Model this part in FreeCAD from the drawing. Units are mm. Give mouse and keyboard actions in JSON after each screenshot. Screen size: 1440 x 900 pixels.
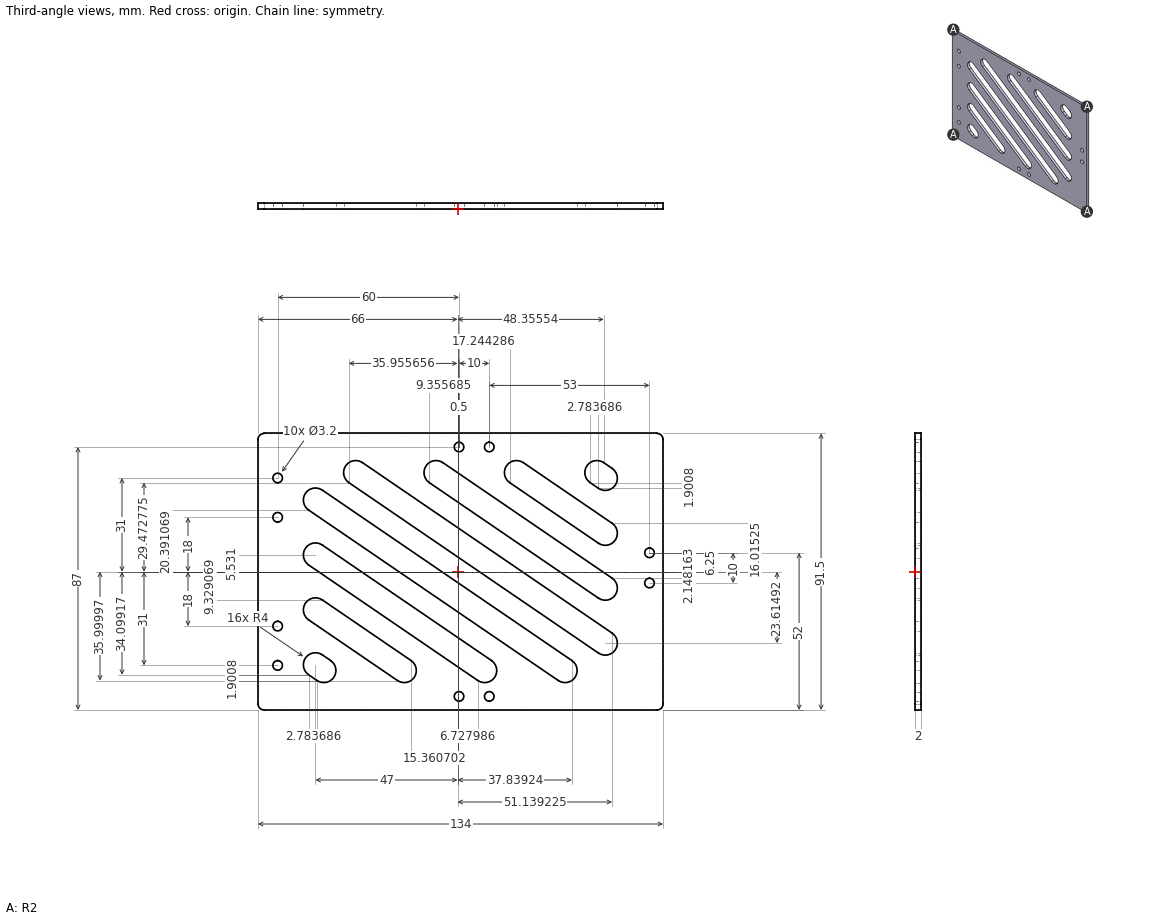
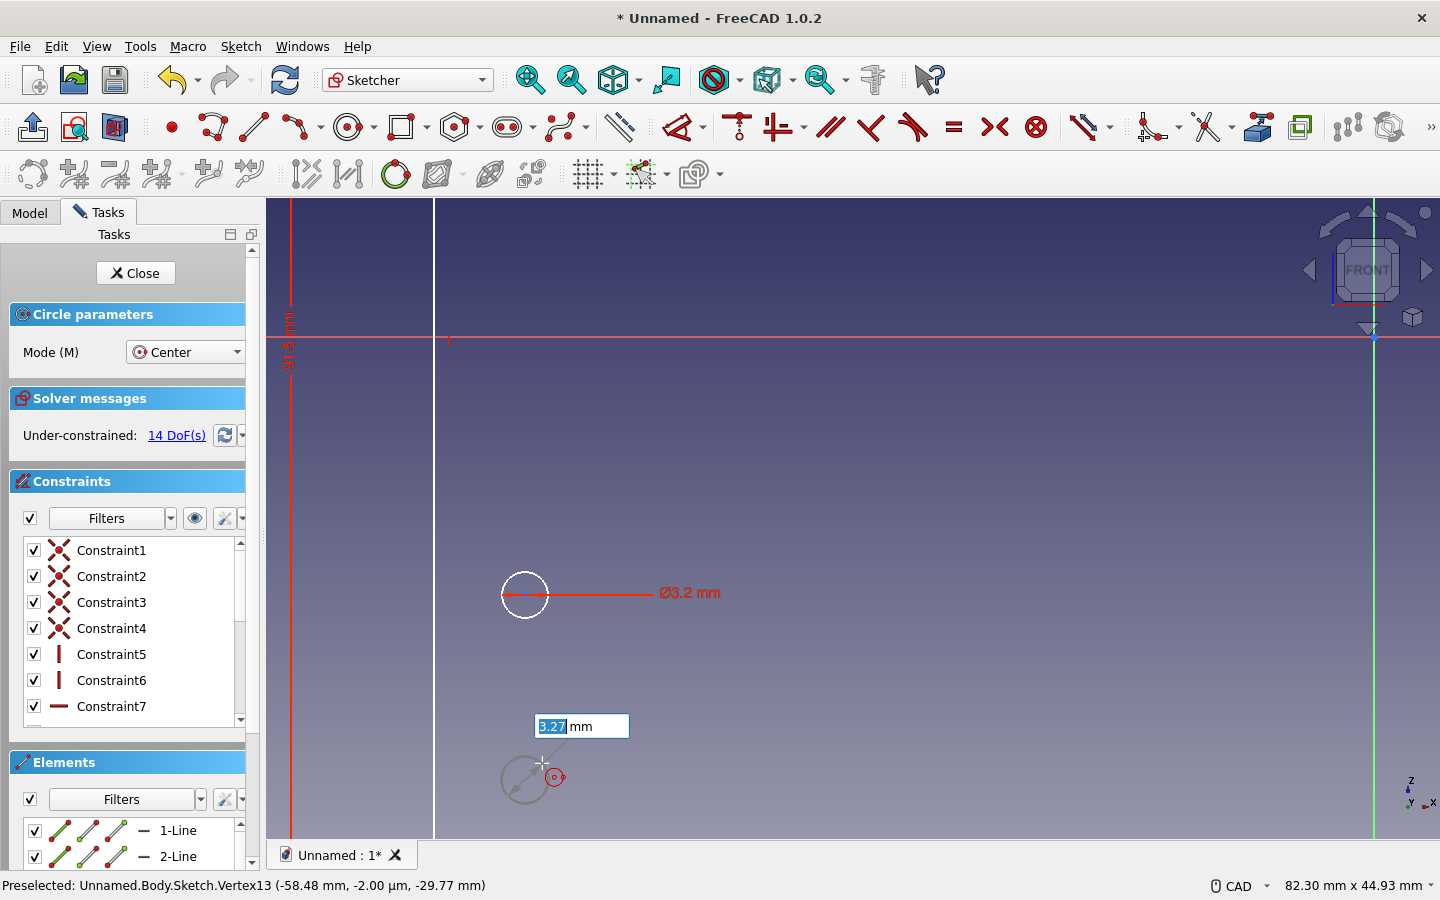
{"action": "type", "text": "3.2"}
{"action": "key", "text": "Return"}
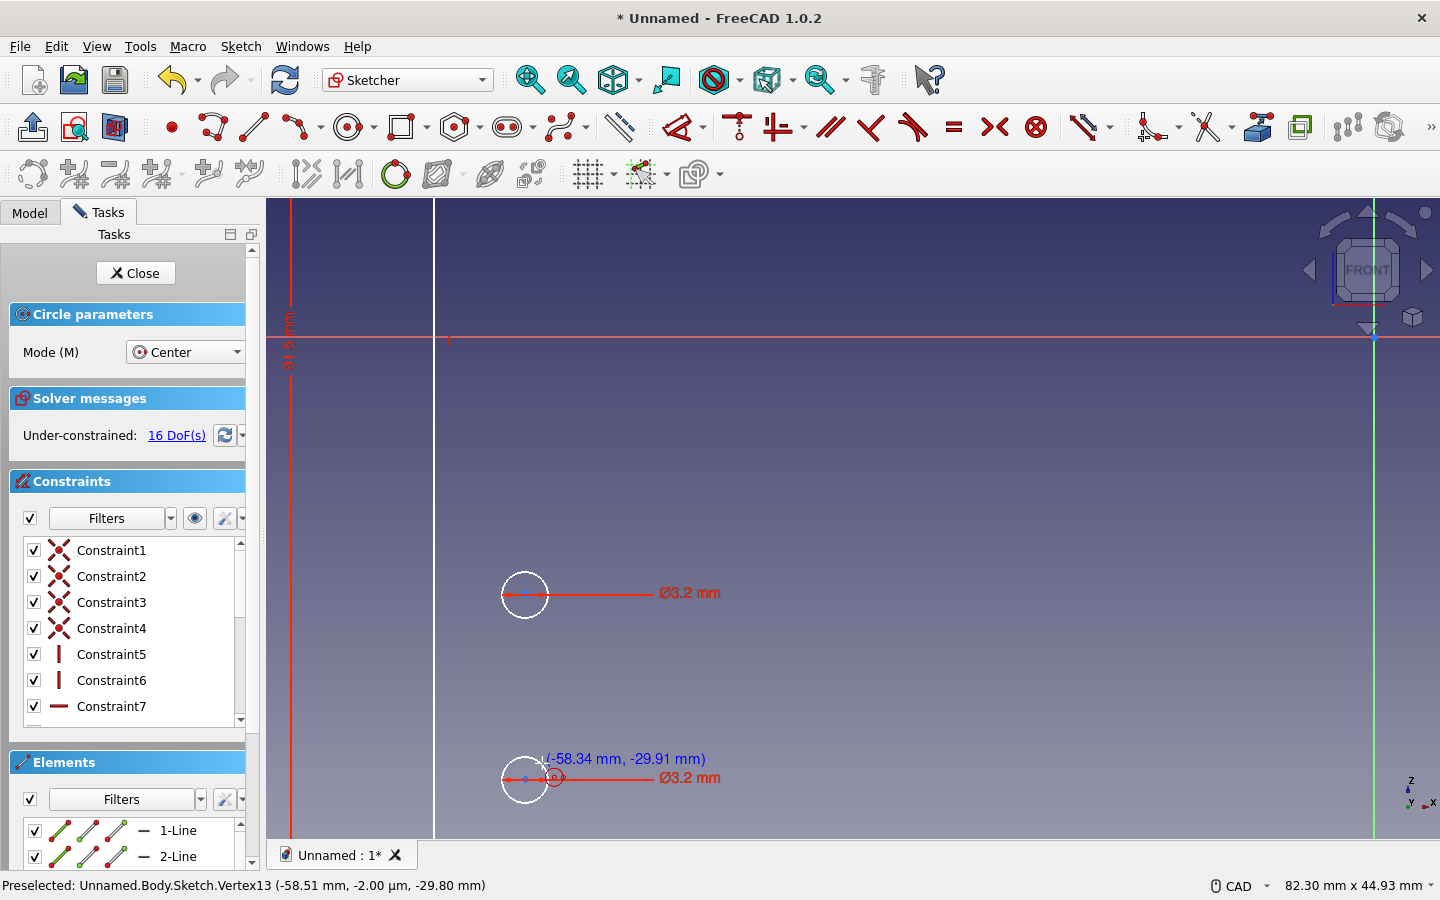
{"action": "scroll", "coordinate": [524, 597], "scroll_direction": "down", "scroll_amount": 6}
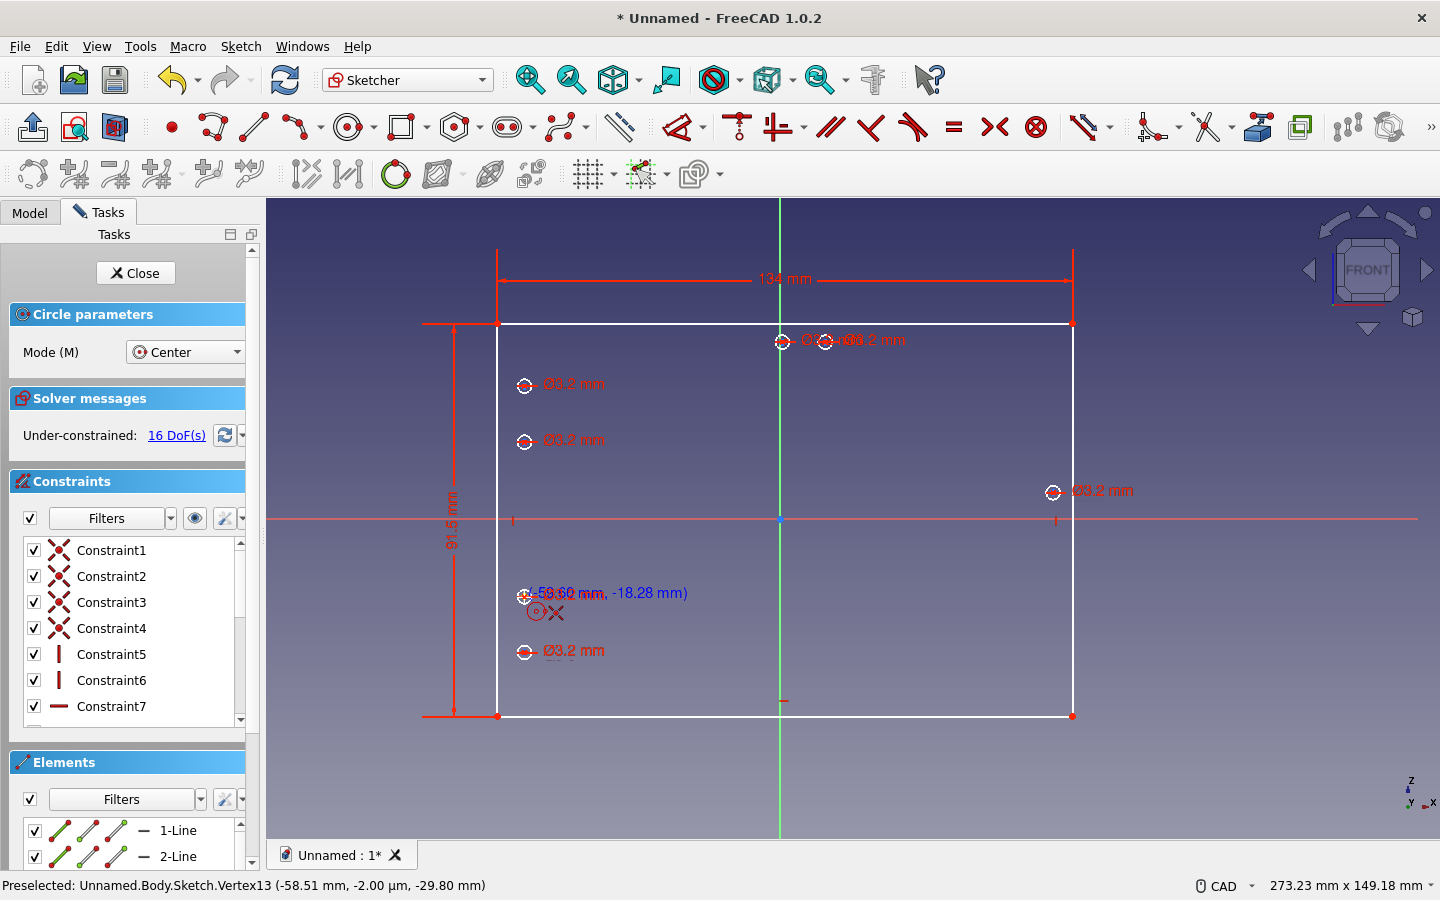
{"action": "scroll", "coordinate": [782, 696], "scroll_direction": "up", "scroll_amount": 11}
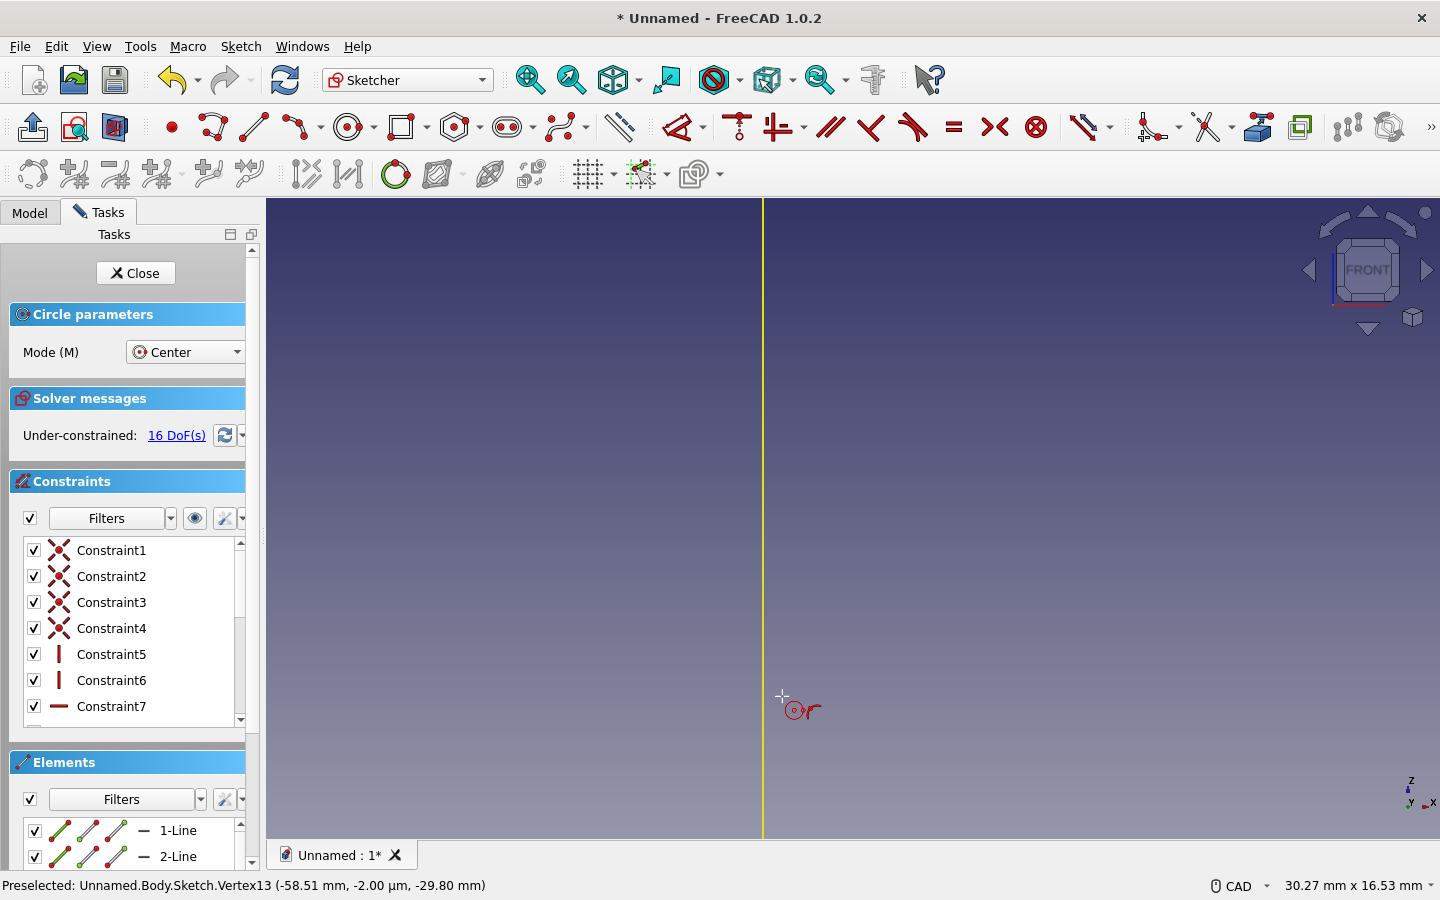
{"action": "left_click", "coordinate": [782, 694]}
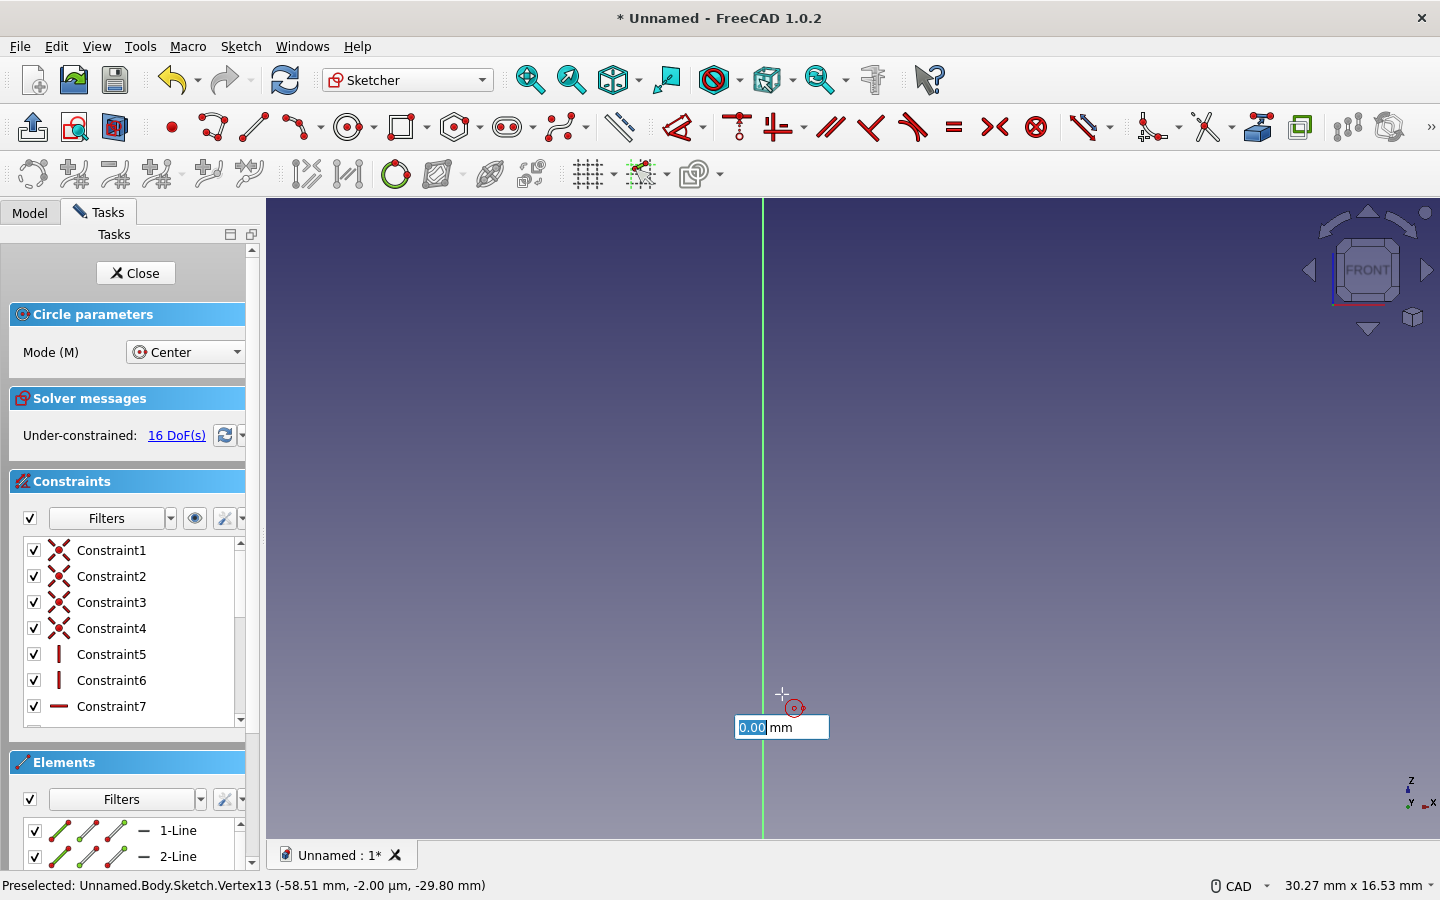
{"action": "scroll", "coordinate": [782, 696], "scroll_direction": "down", "scroll_amount": 11}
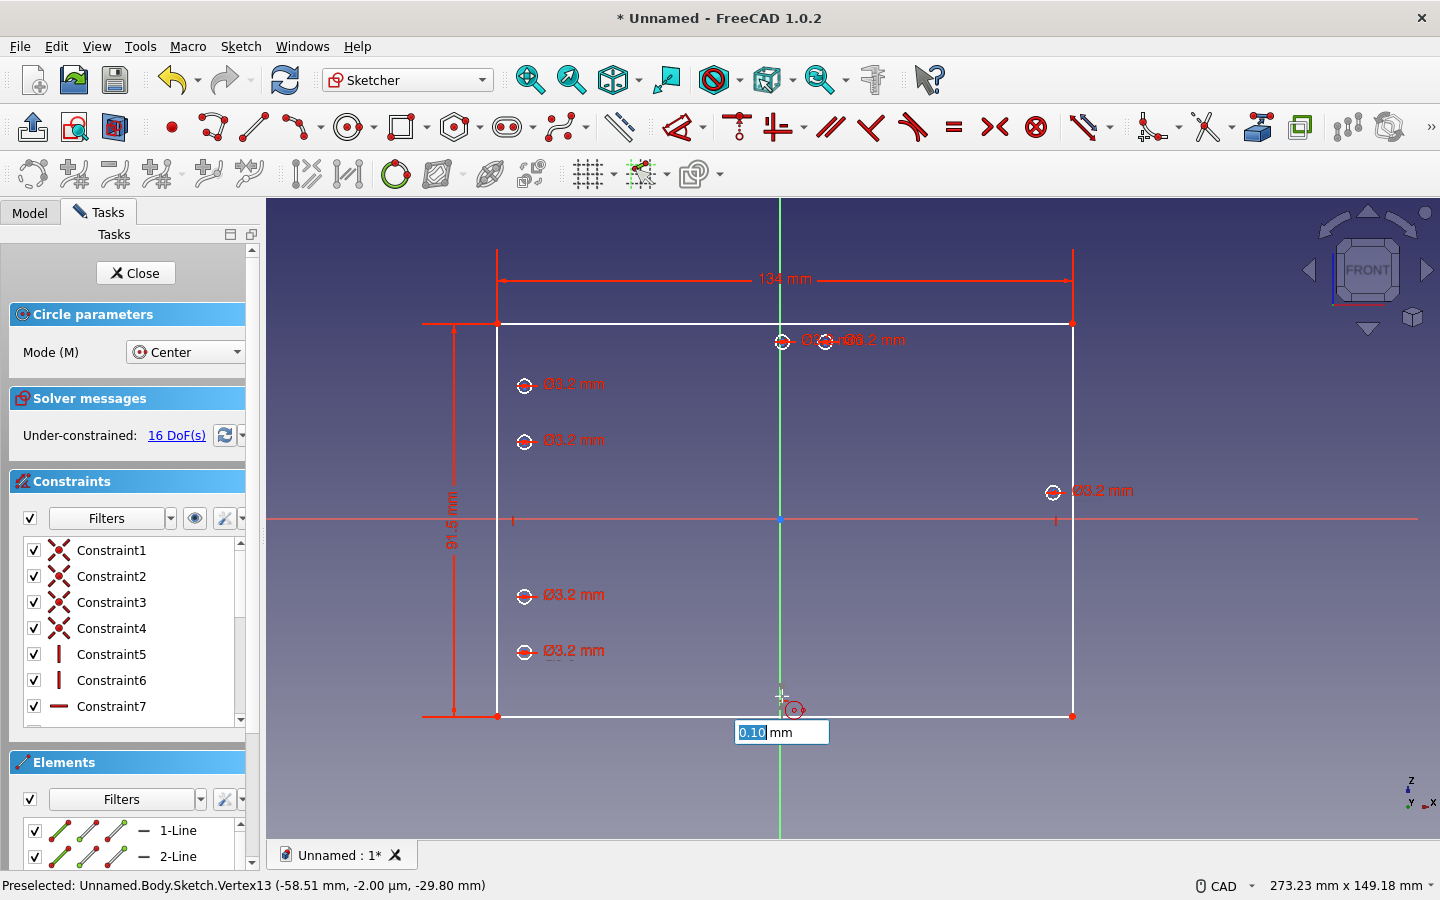
{"action": "scroll", "coordinate": [787, 692], "scroll_direction": "up", "scroll_amount": 5}
{"action": "mouse_move", "coordinate": [787, 690]}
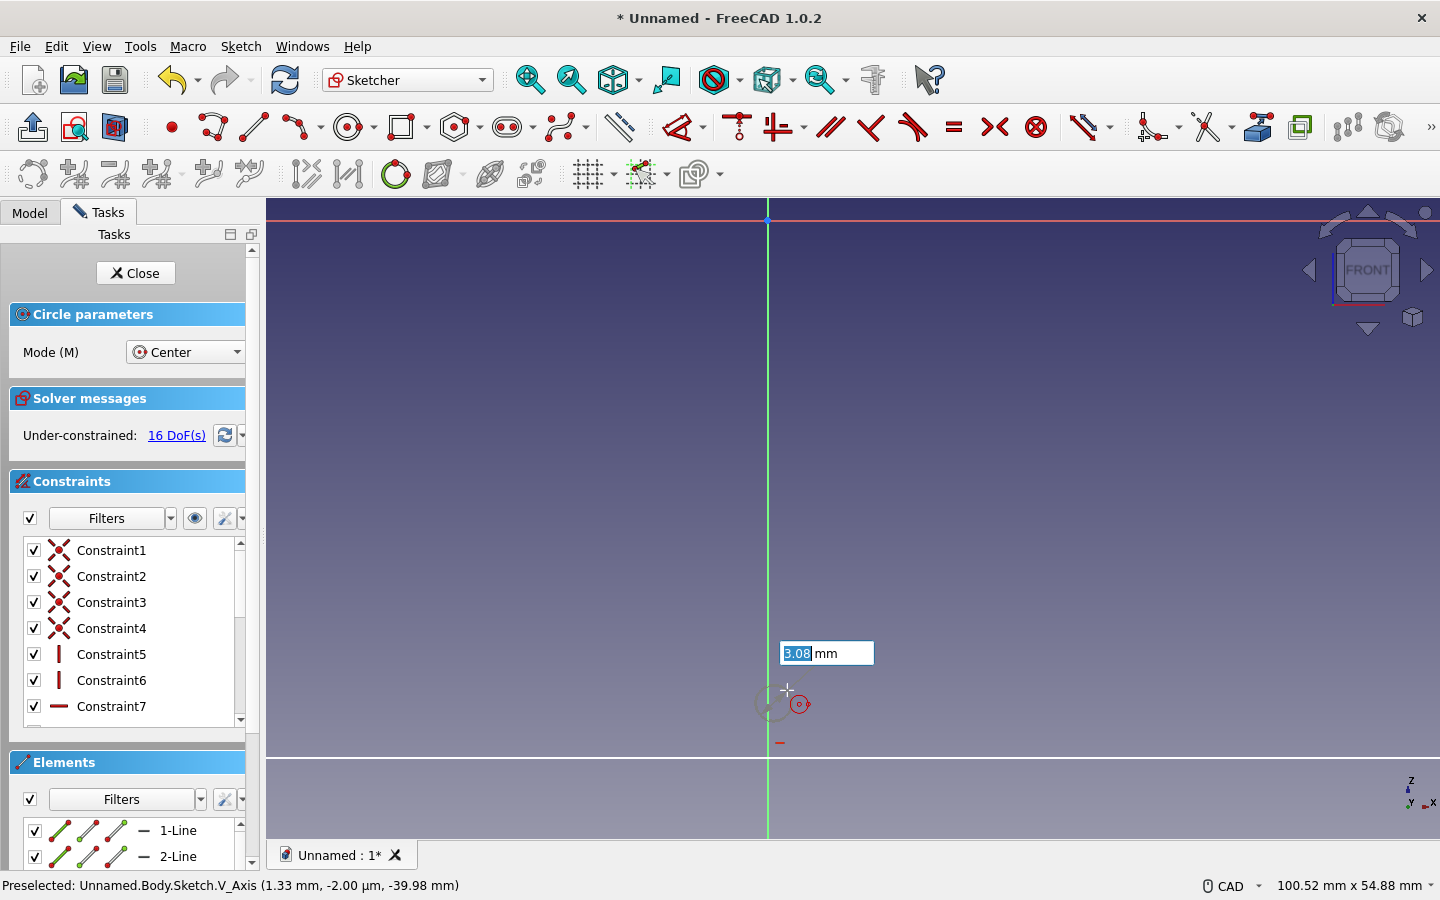
{"action": "type", "text": "3.2"}
{"action": "key", "text": "Return"}